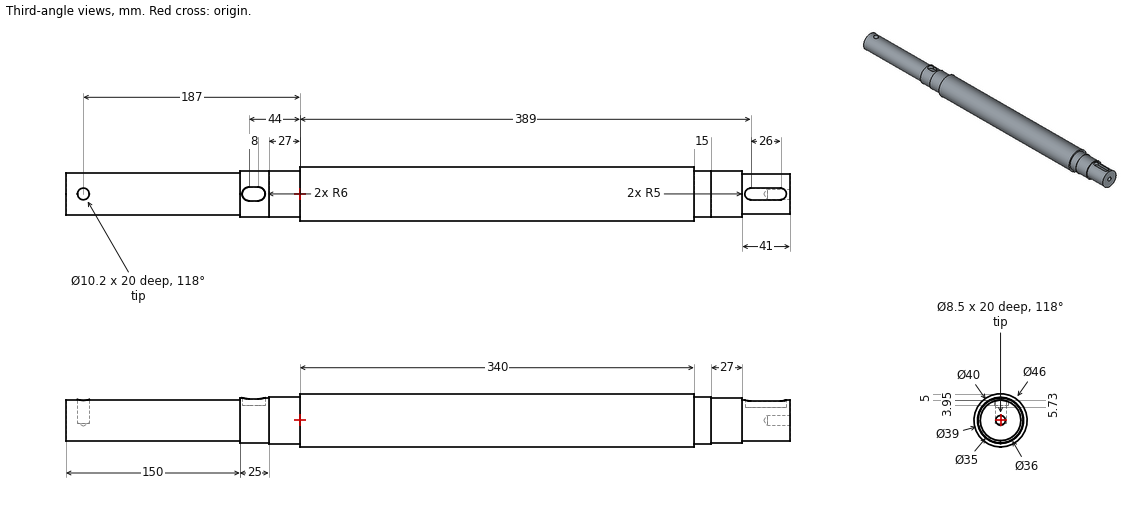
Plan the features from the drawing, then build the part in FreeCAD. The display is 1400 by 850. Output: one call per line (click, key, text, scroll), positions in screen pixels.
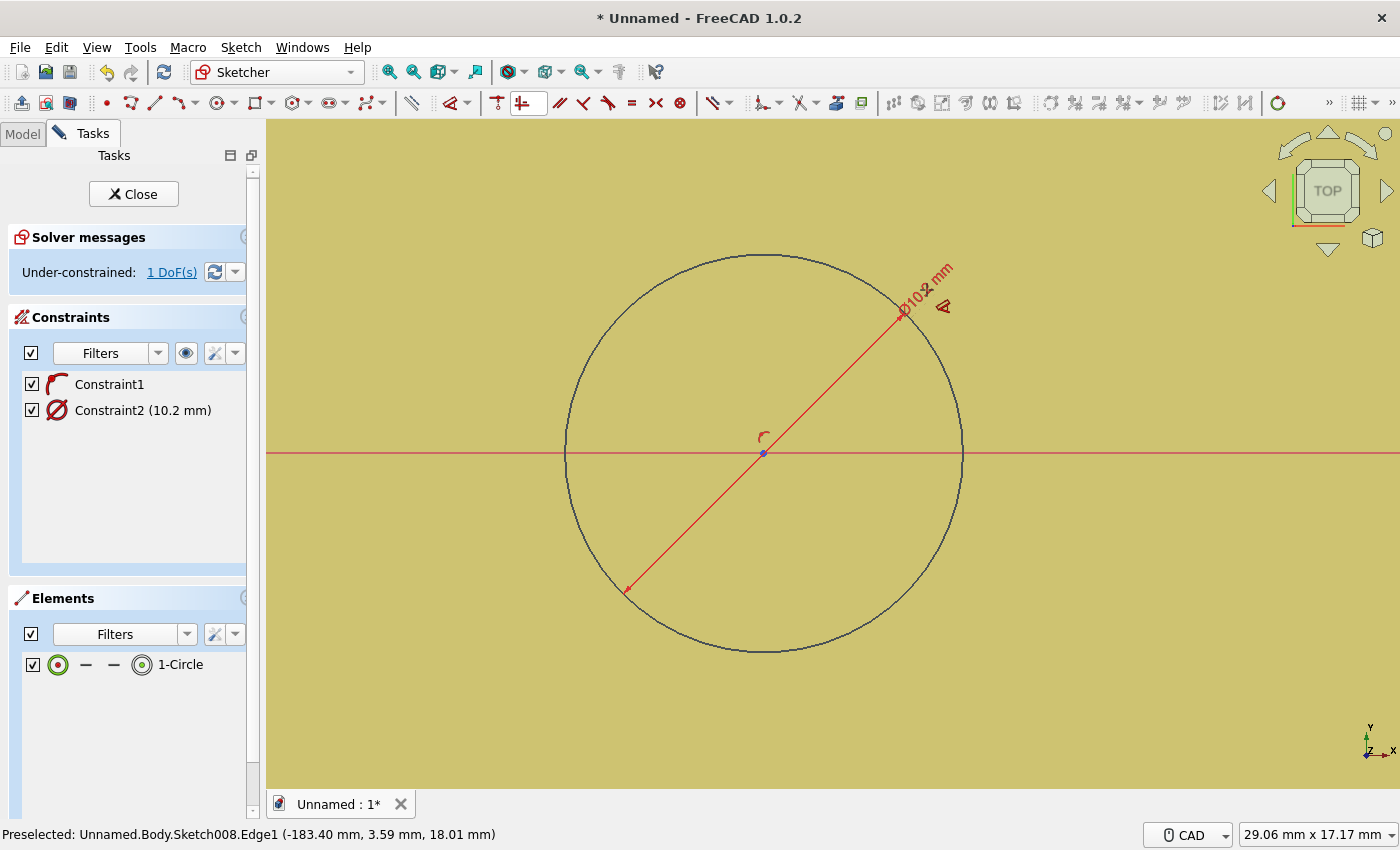
click(764, 453)
click(999, 487)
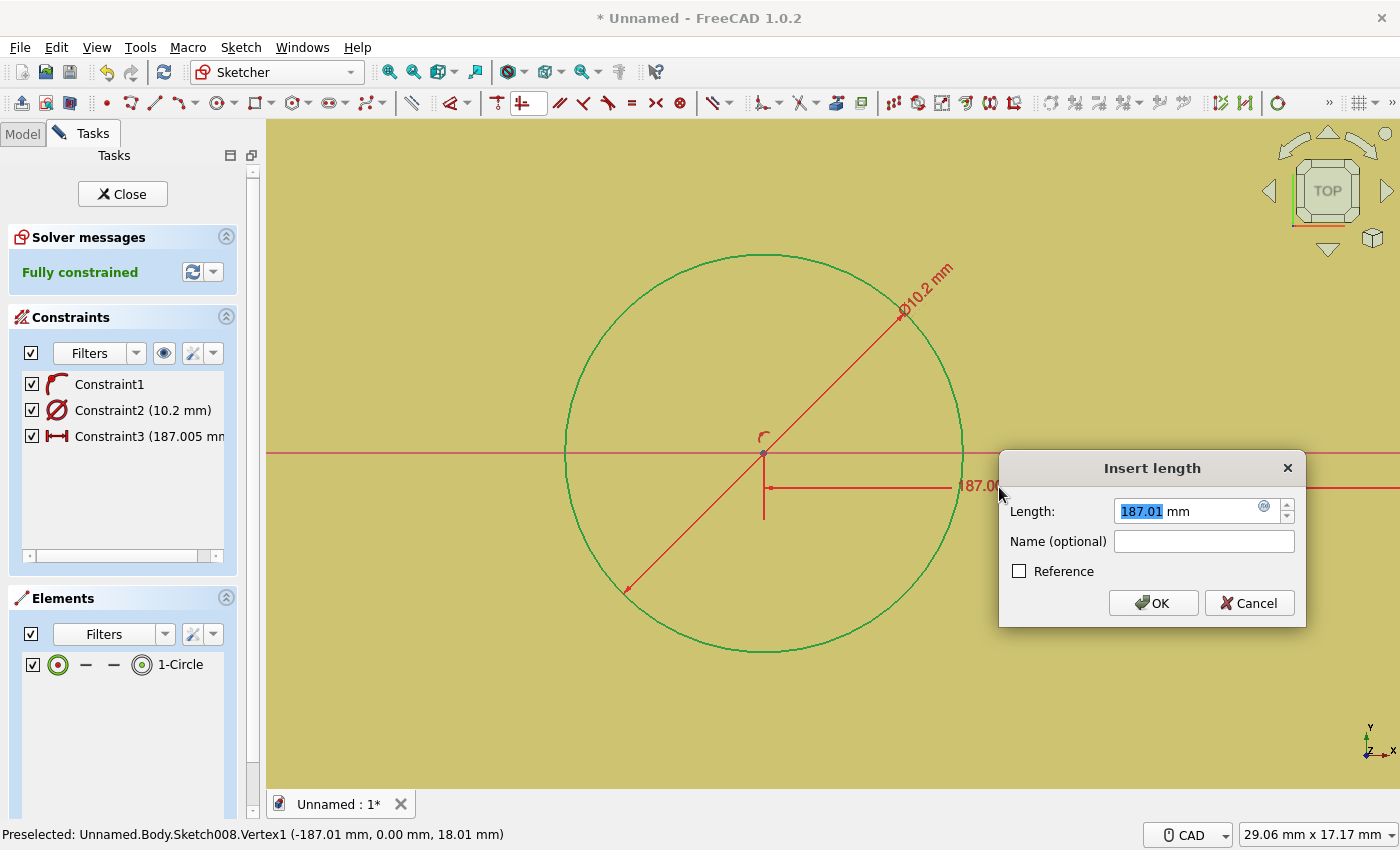
text(187)
key(Return)
key(Escape)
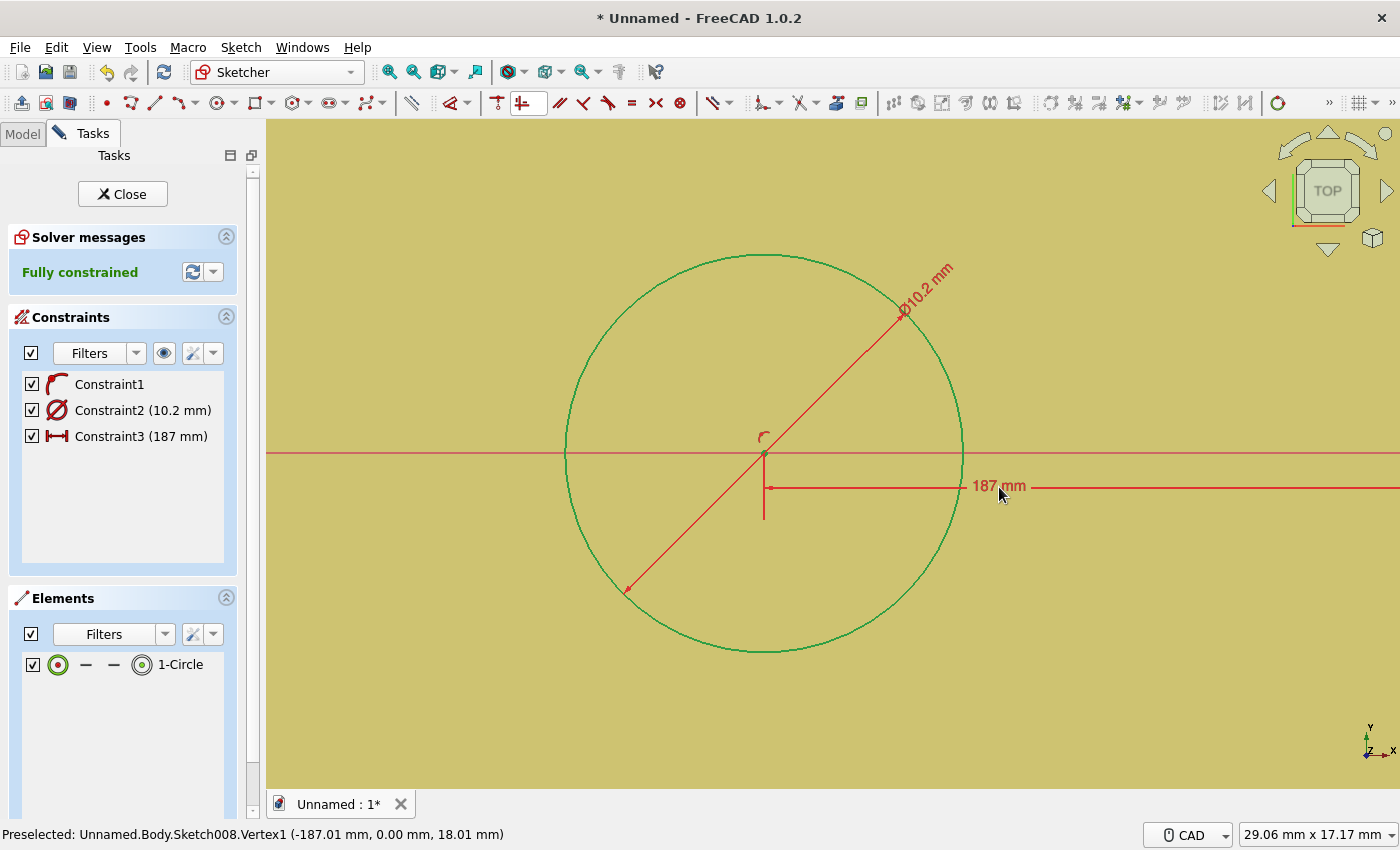
click(123, 194)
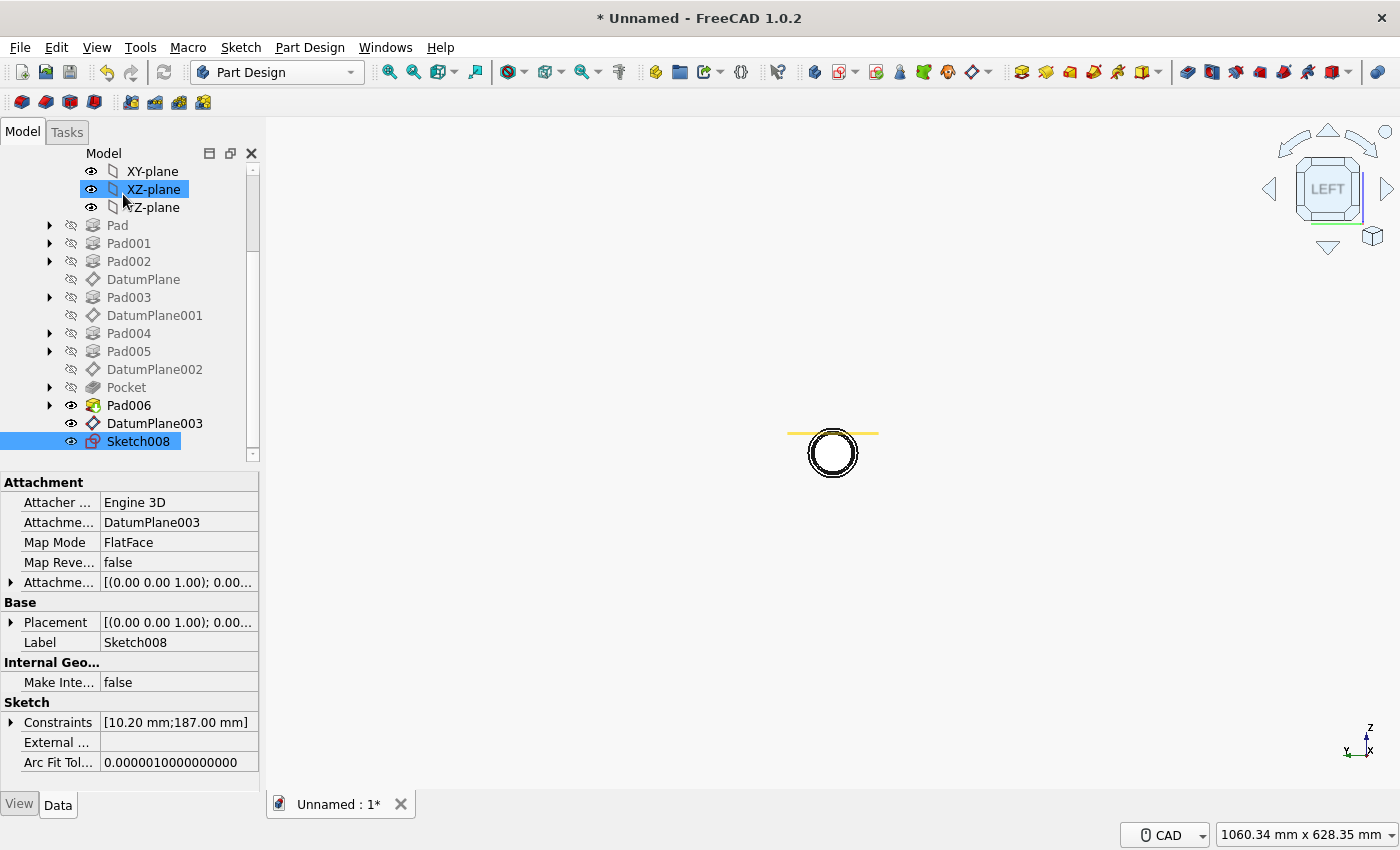
click(1212, 72)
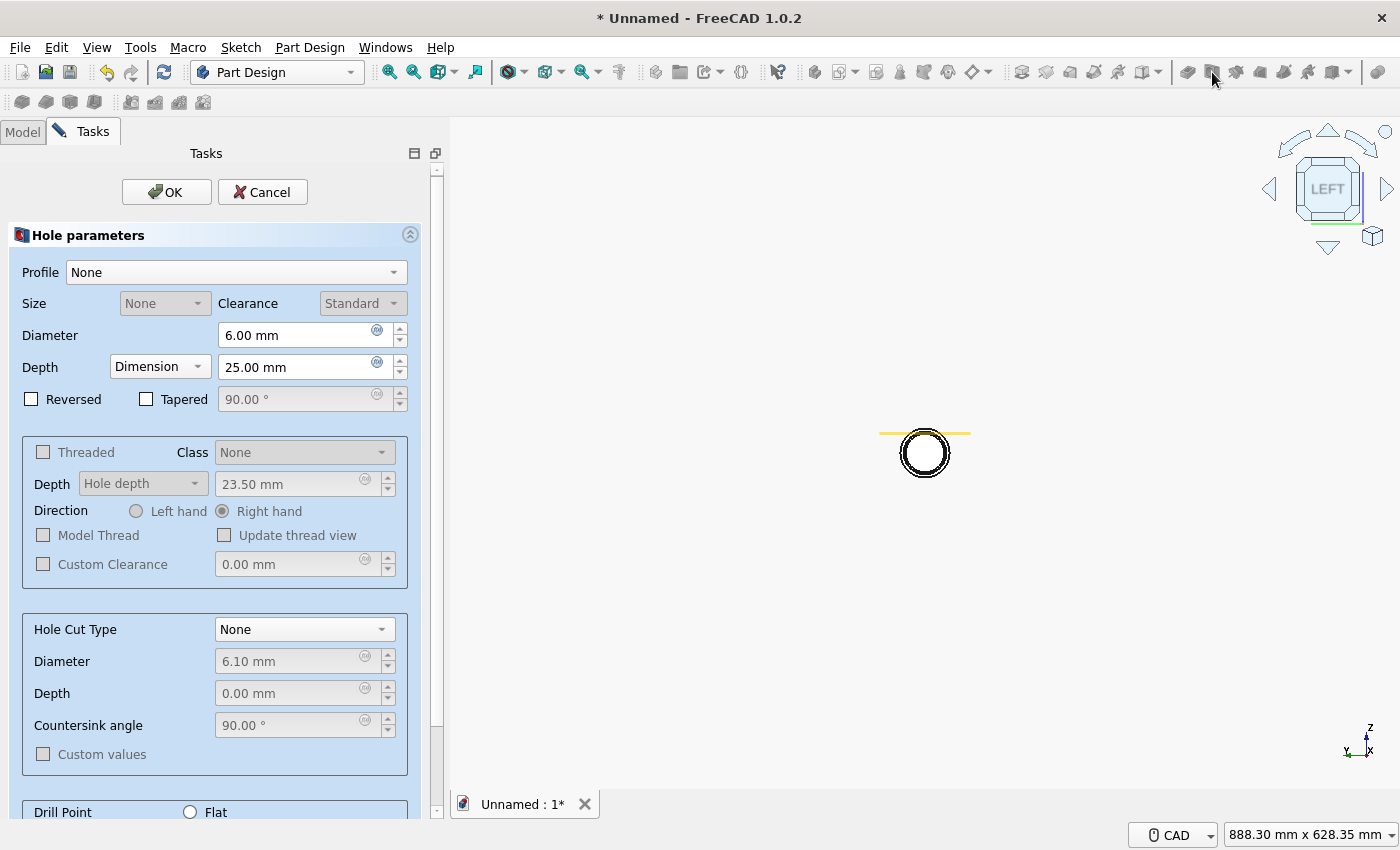
triple_click(305, 335)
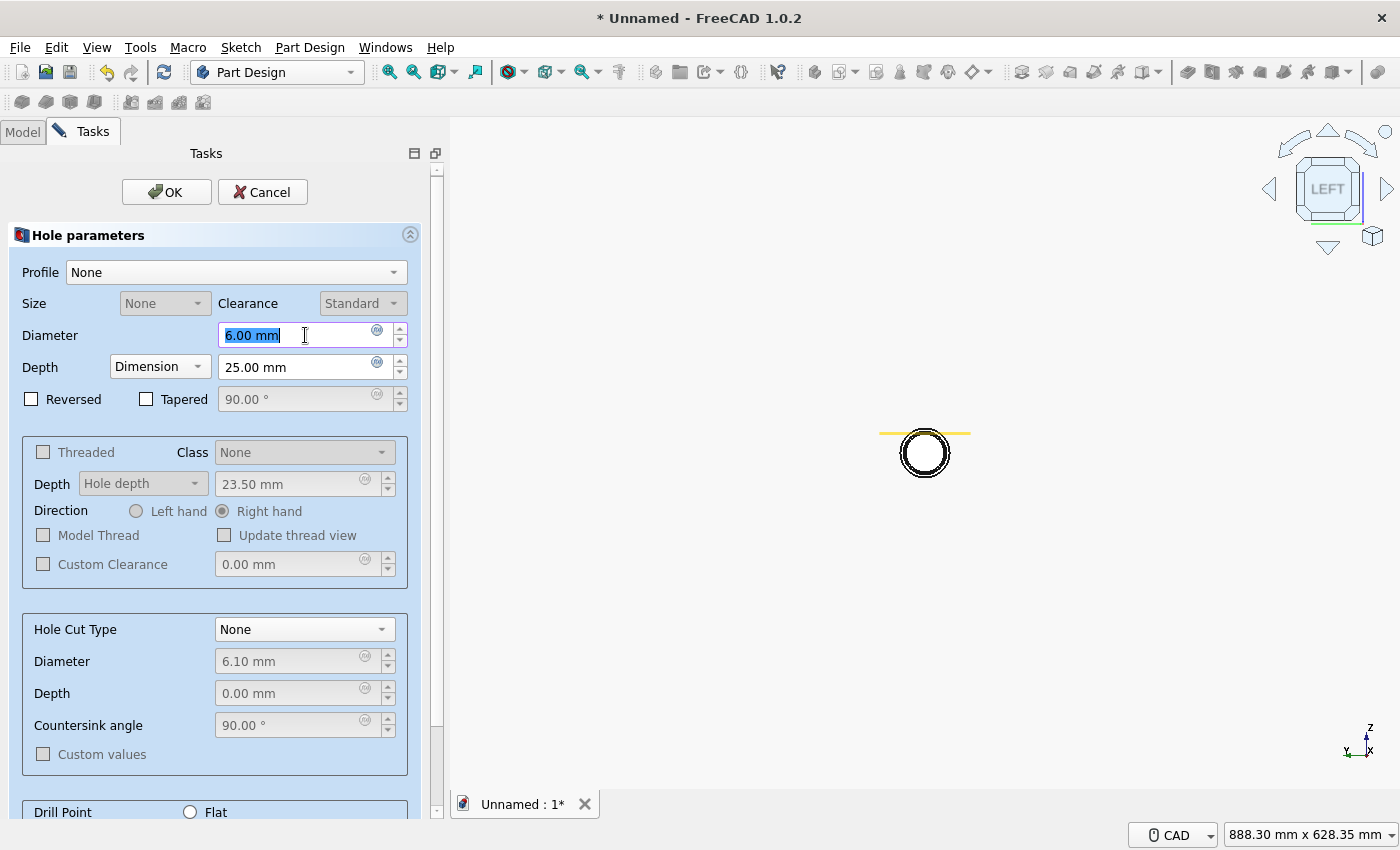
text(10.2)
key(Tab)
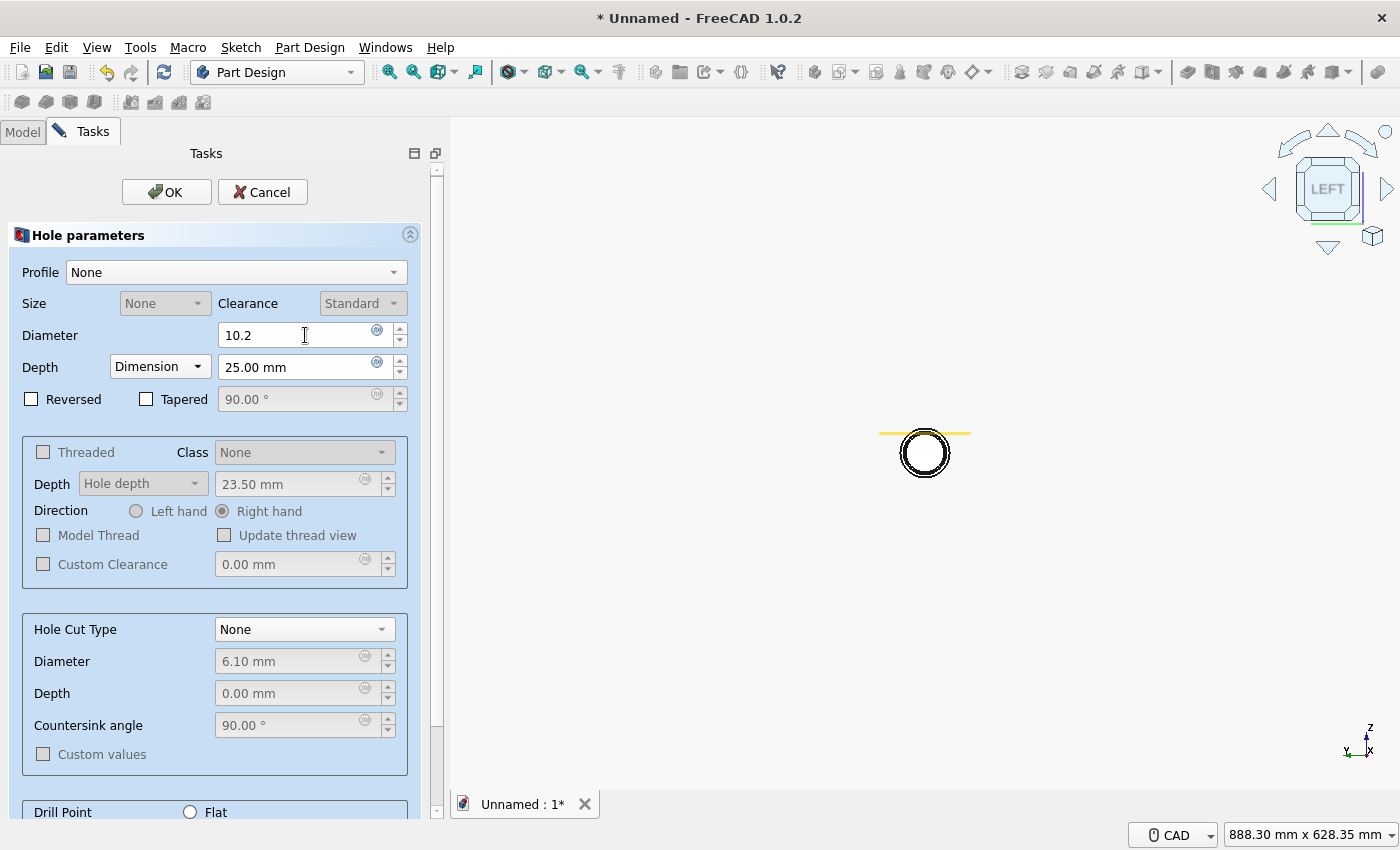
triple_click(305, 367)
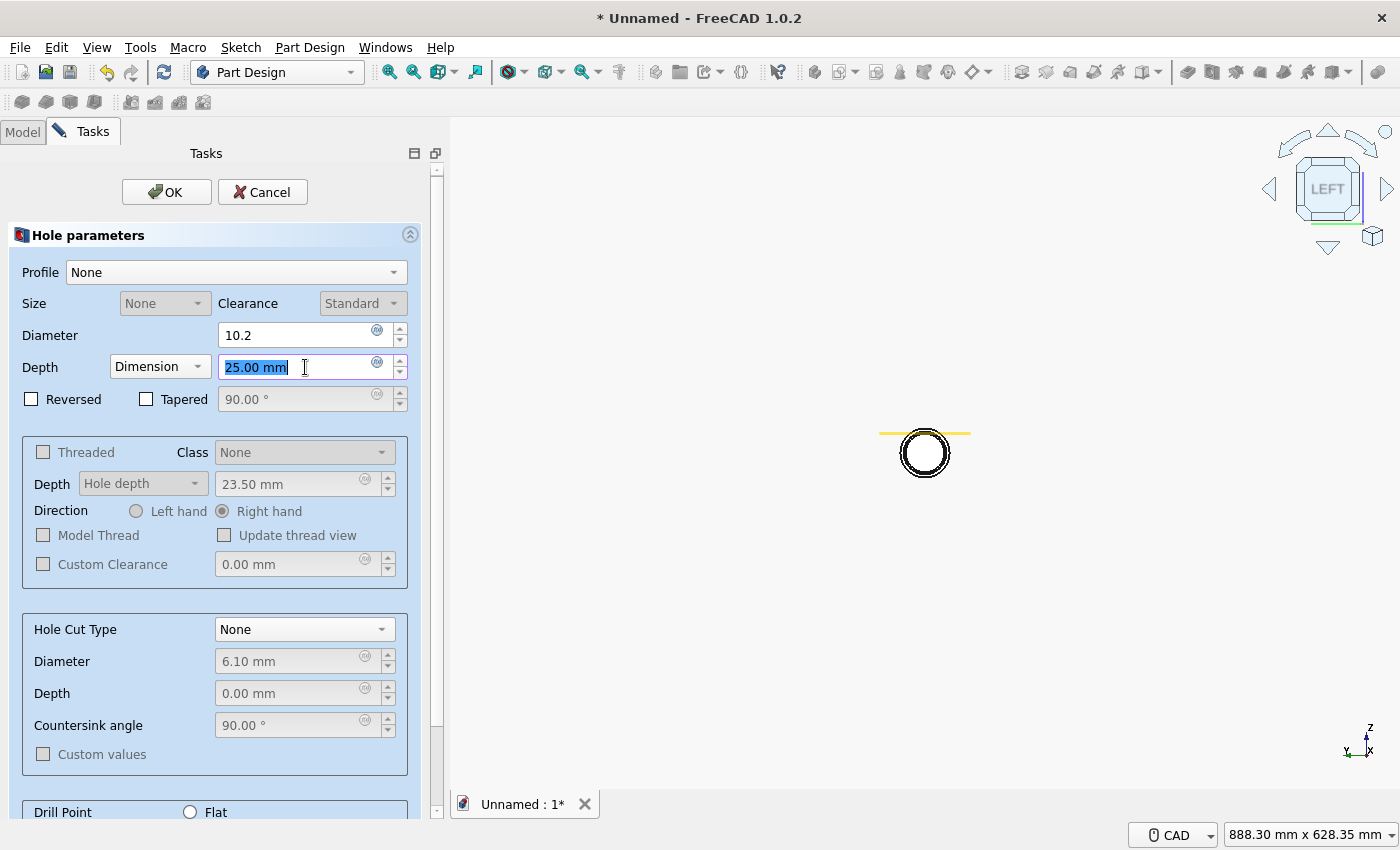
text(20)
key(Tab)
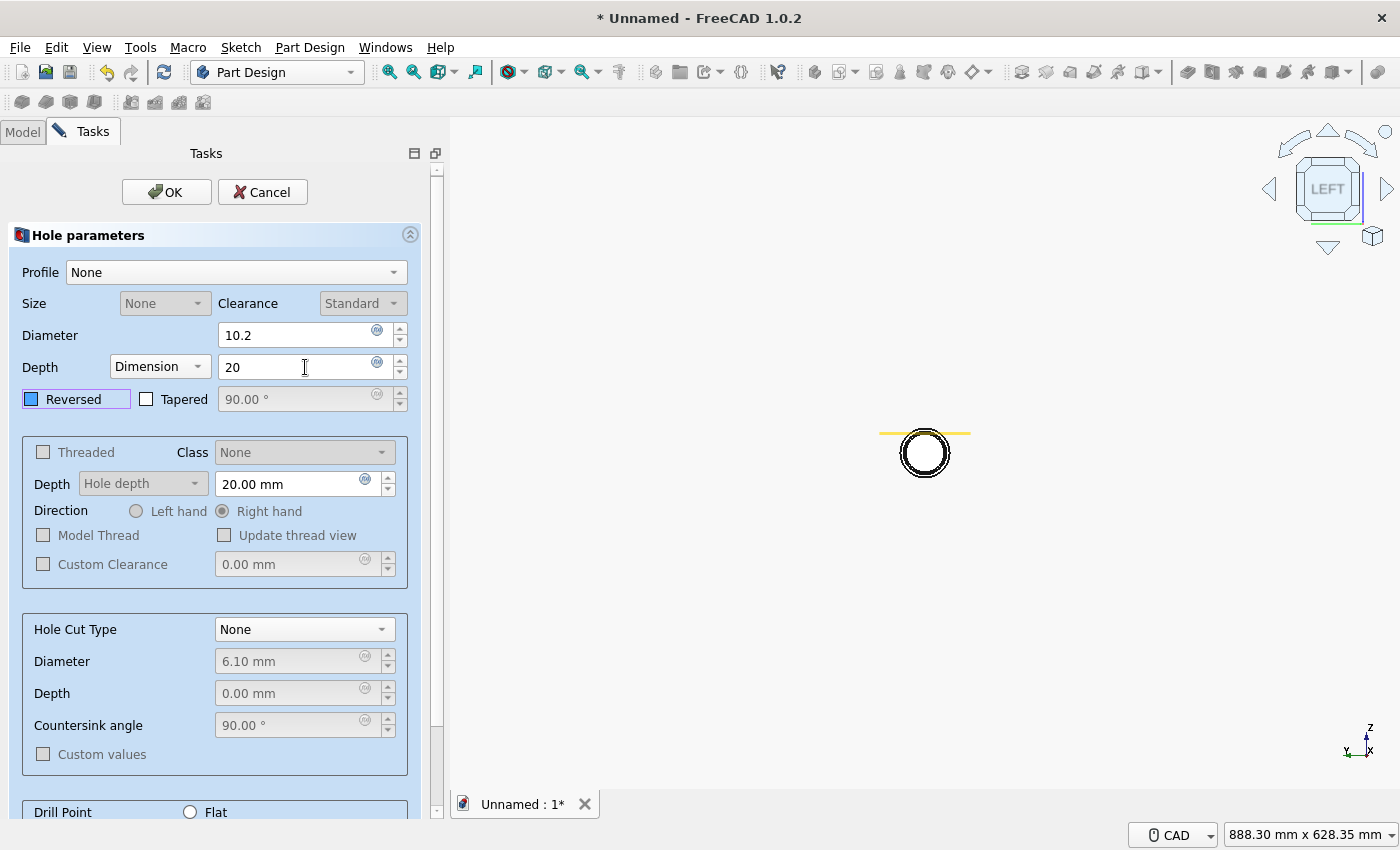
click(167, 192)